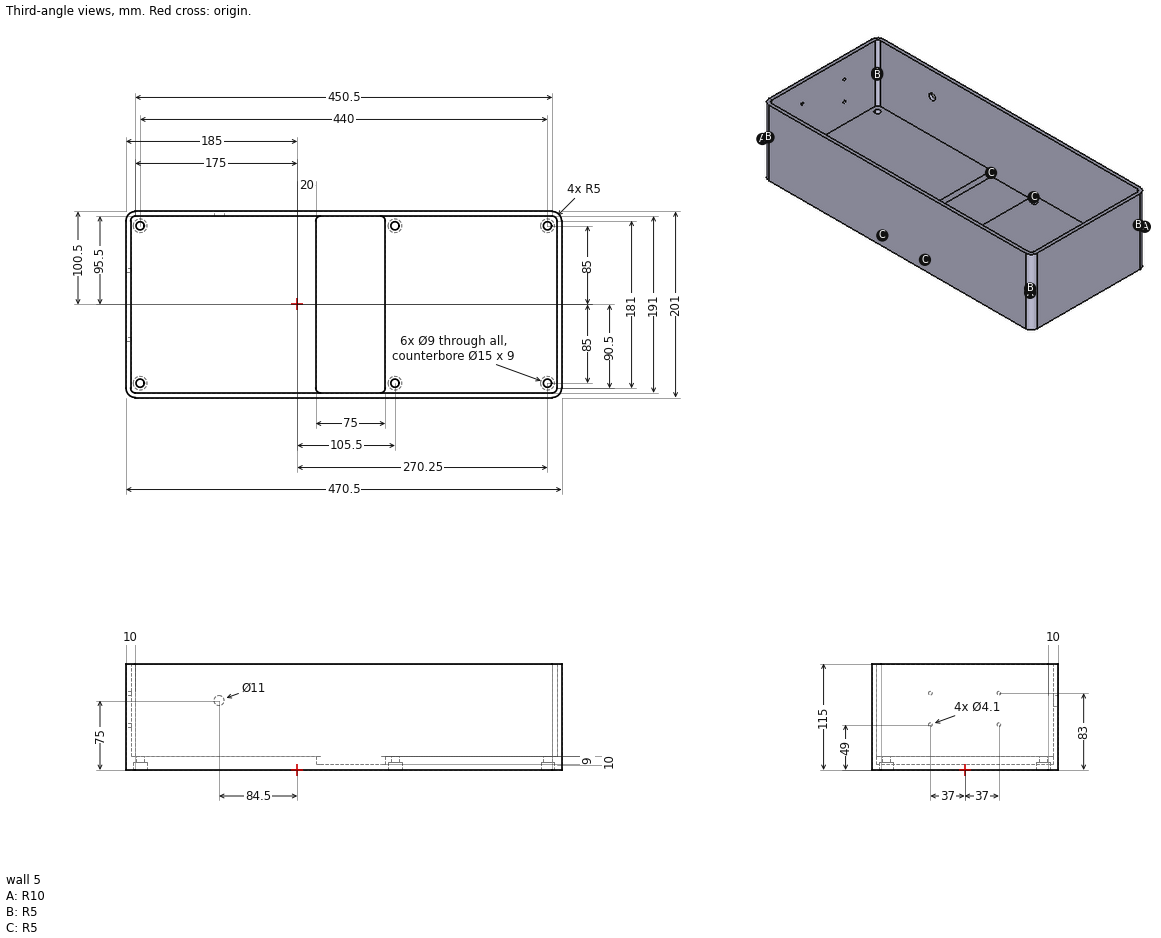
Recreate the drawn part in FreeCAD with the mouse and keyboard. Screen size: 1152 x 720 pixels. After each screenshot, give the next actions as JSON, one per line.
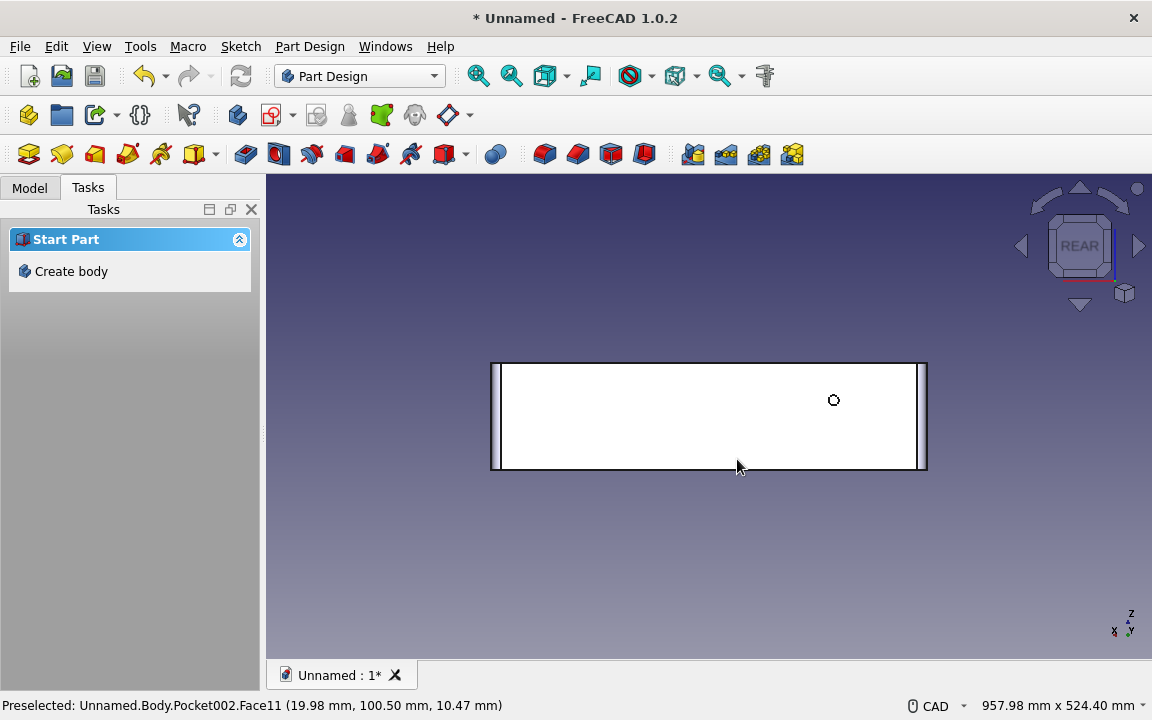
{"action": "key", "text": "6"}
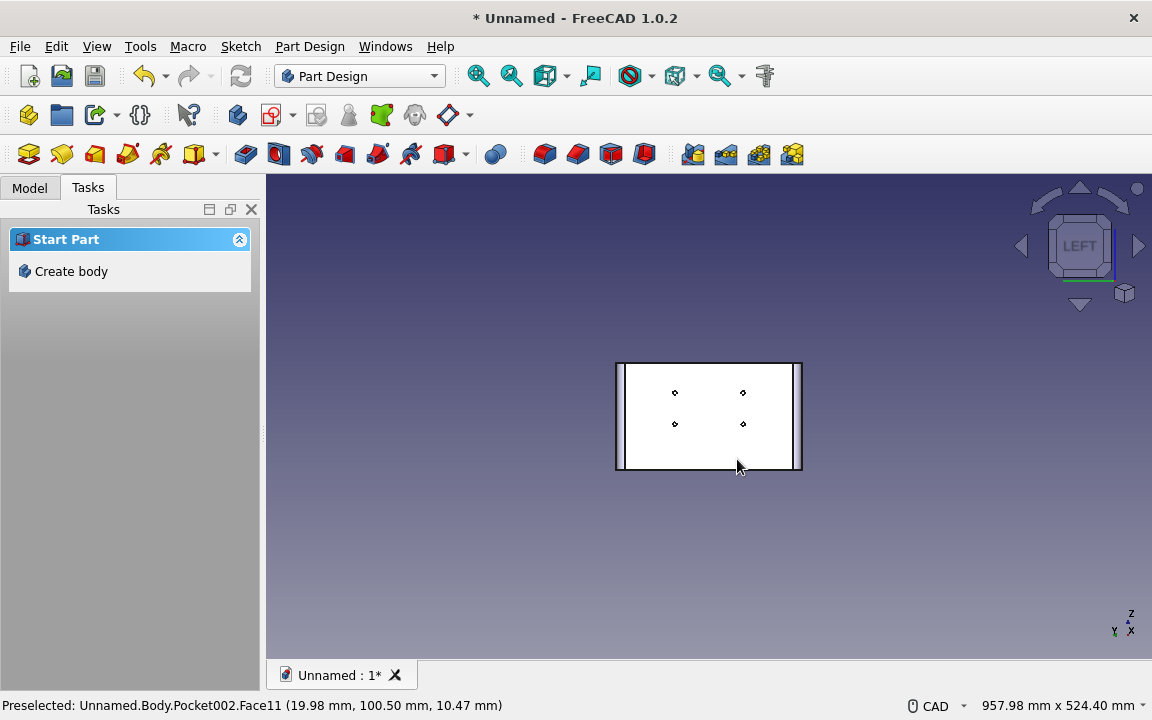
{"action": "key", "text": "v f"}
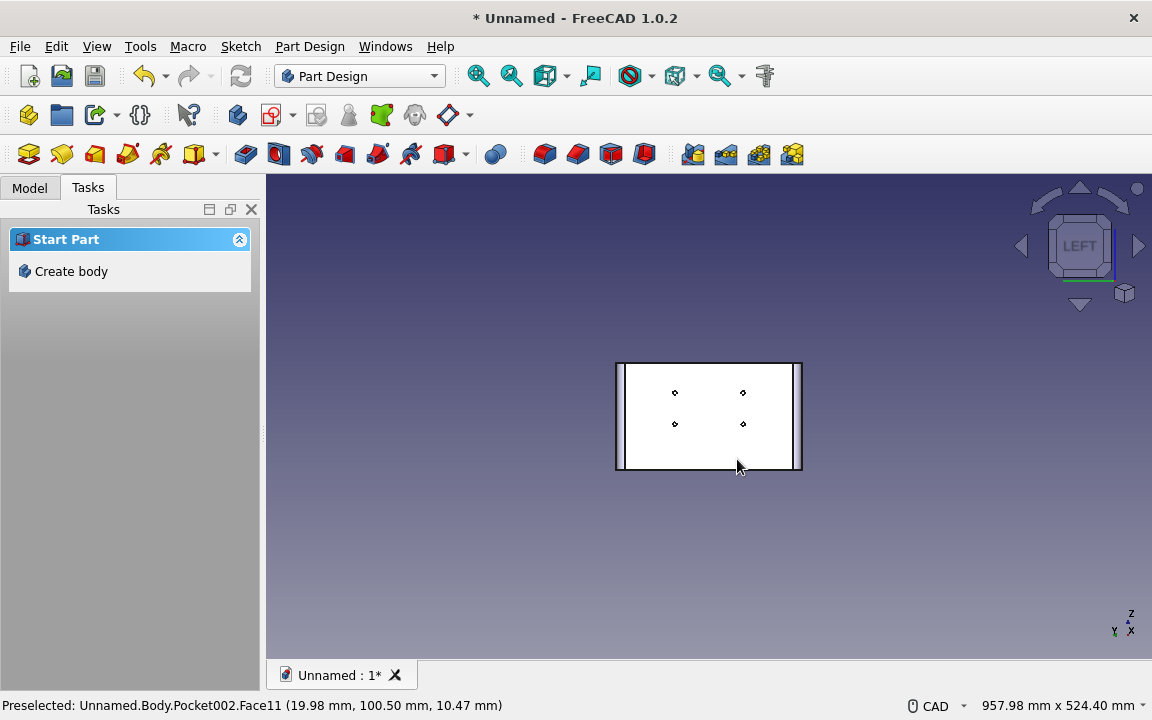
{"action": "scroll", "coordinate": [797, 459], "scroll_direction": "up", "scroll_amount": 8}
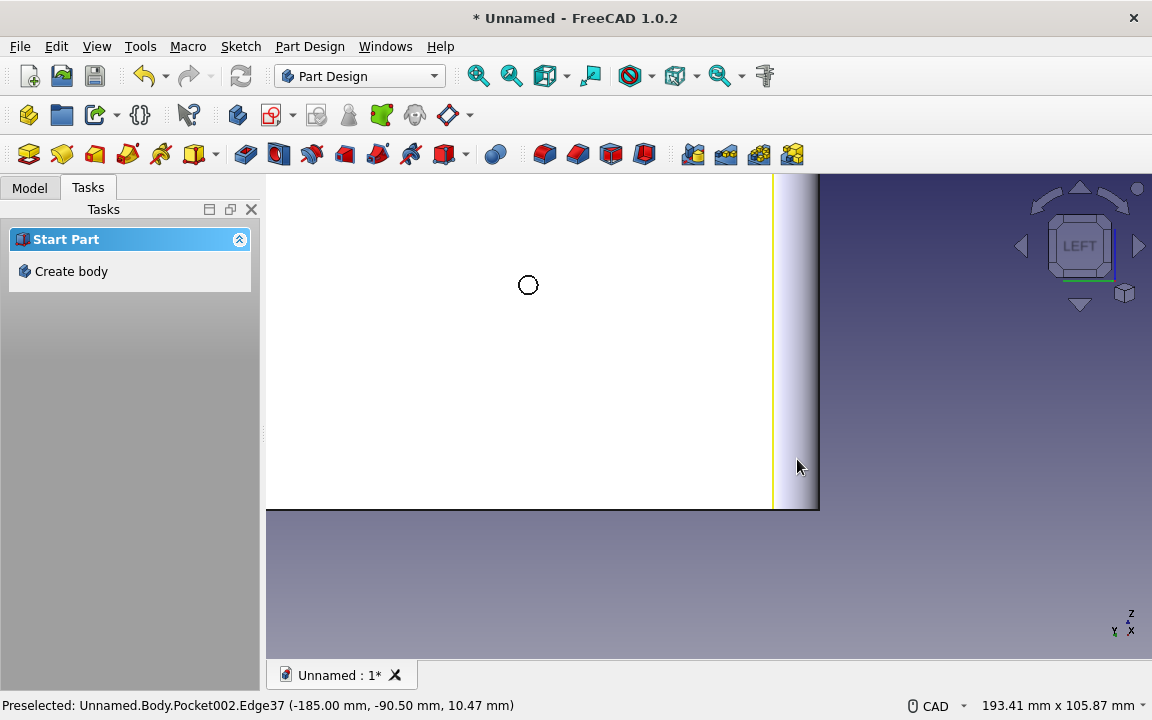
{"action": "key", "text": "v f"}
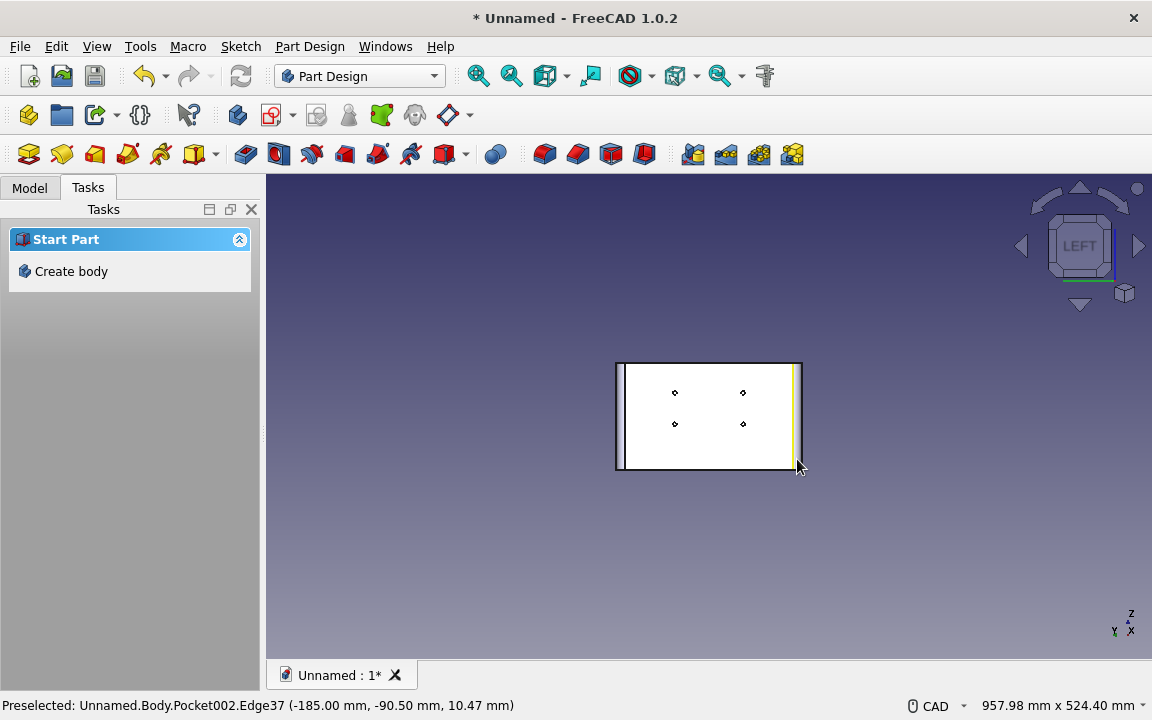
{"action": "key", "text": "v 3"}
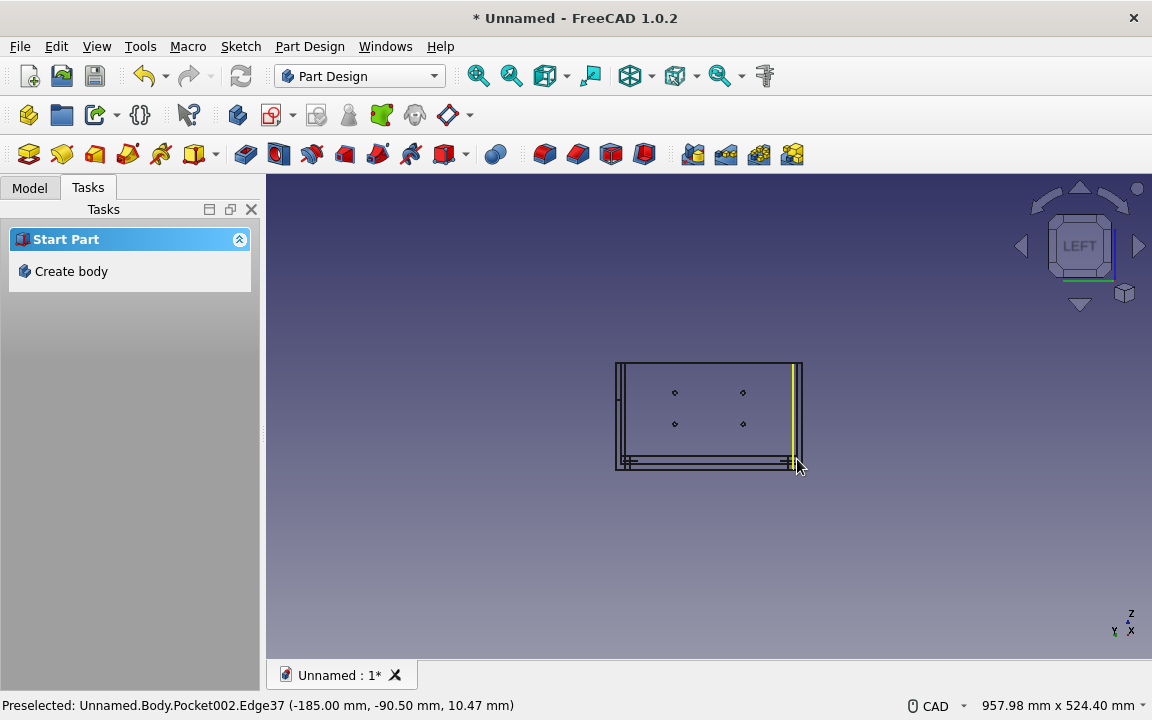
{"action": "key", "text": "0"}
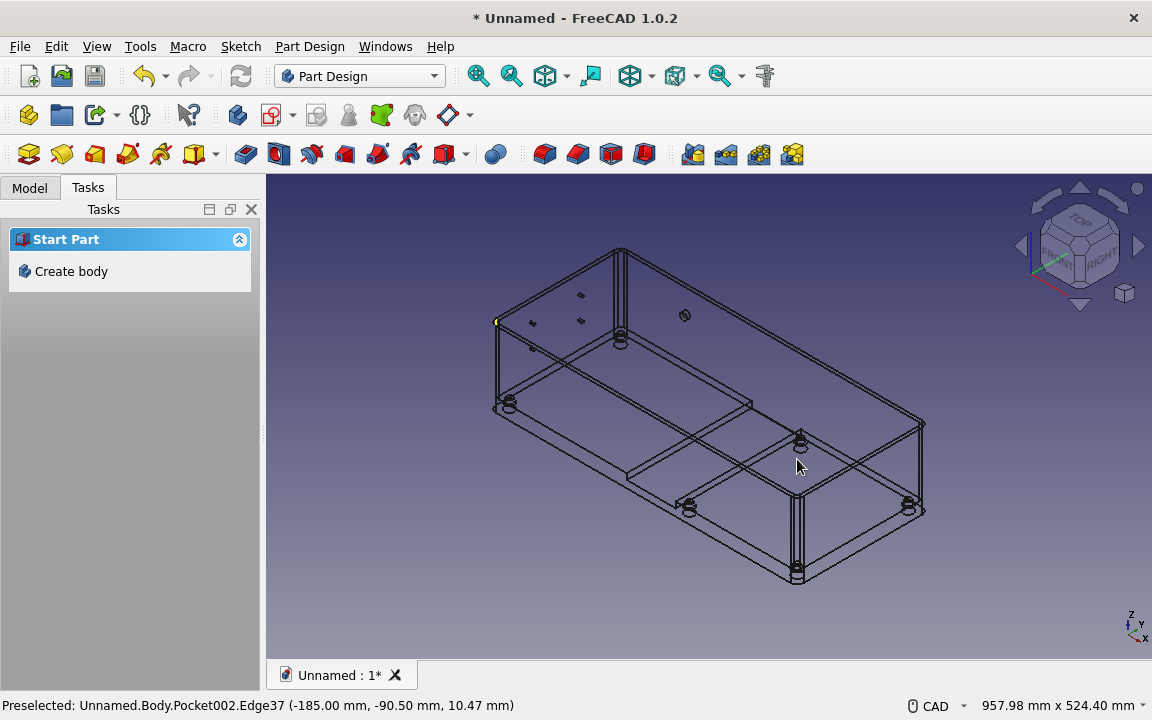
{"action": "scroll", "coordinate": [627, 476], "scroll_direction": "up", "scroll_amount": 8}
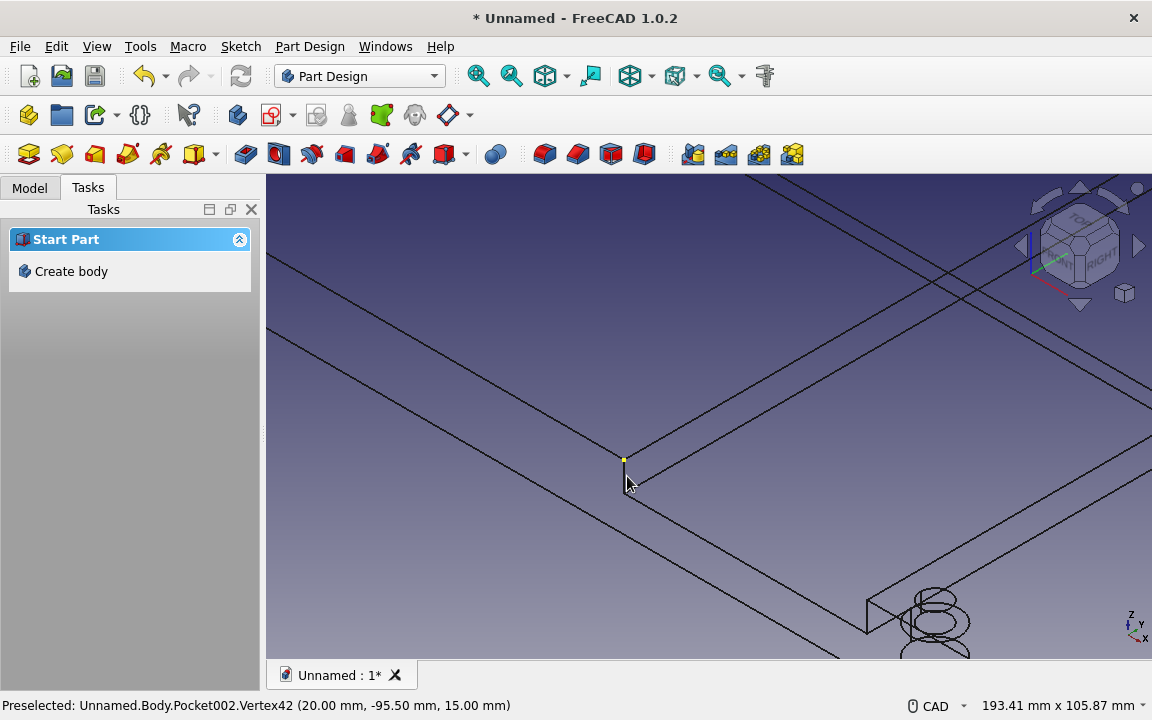
{"action": "left_click", "coordinate": [624, 476]}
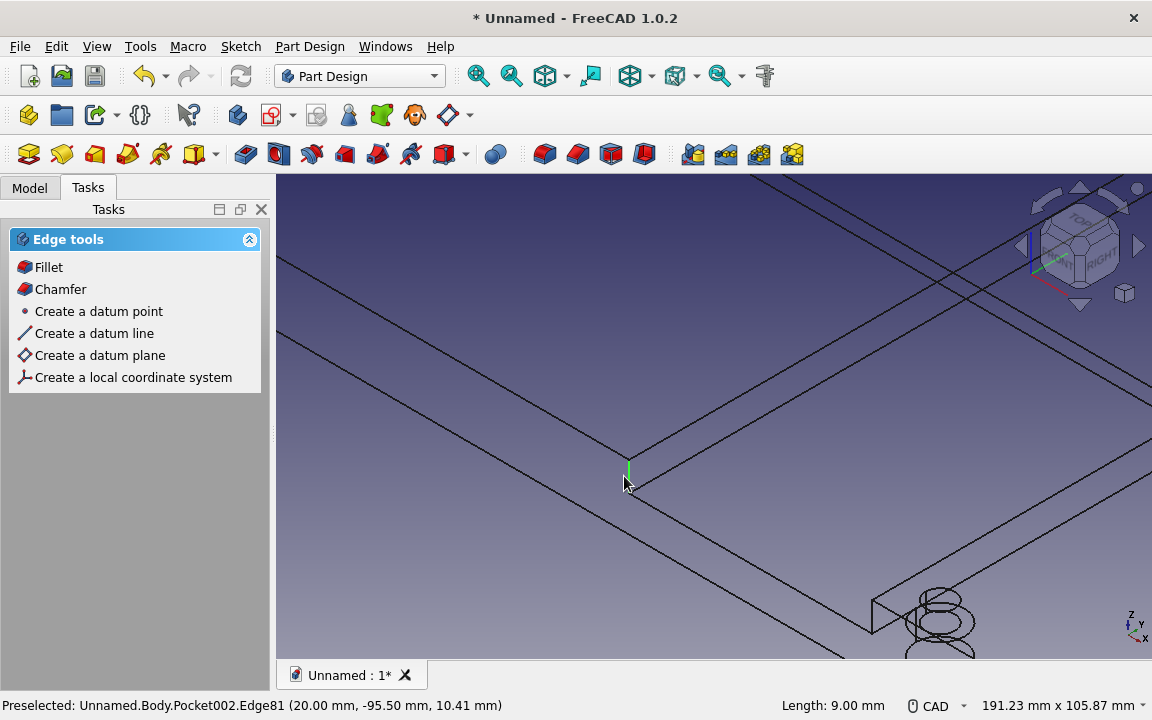
{"action": "left_click", "coordinate": [872, 616], "text": "ctrl"}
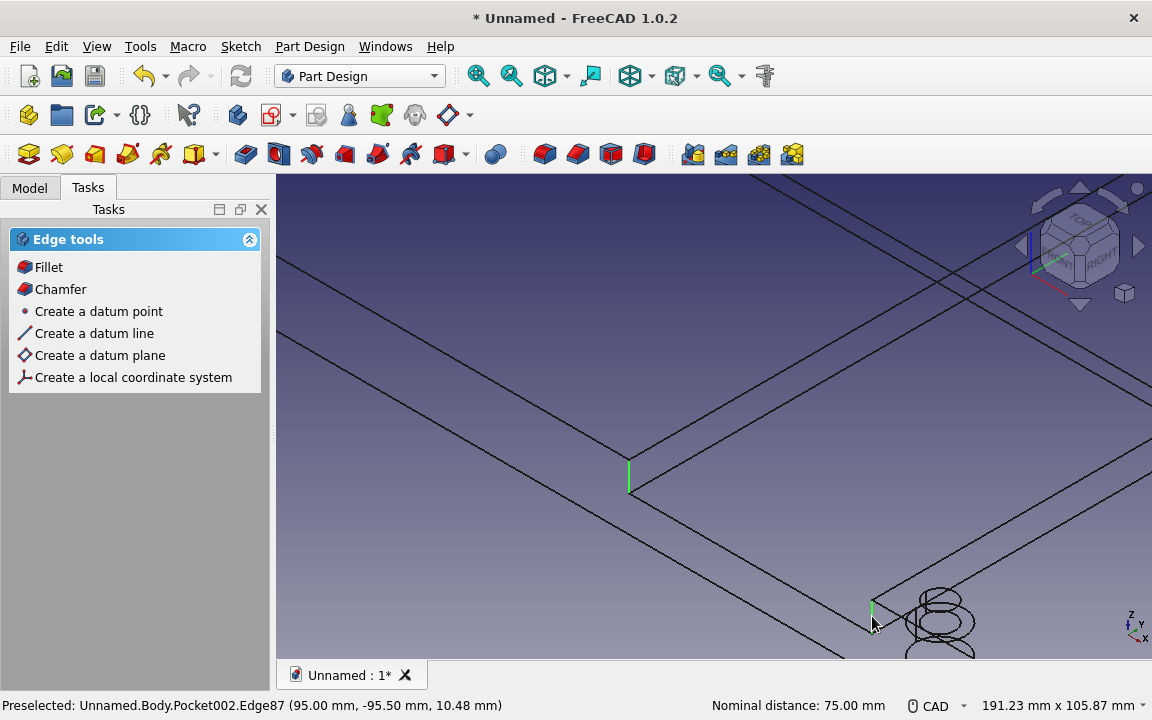
{"action": "key", "text": "v f"}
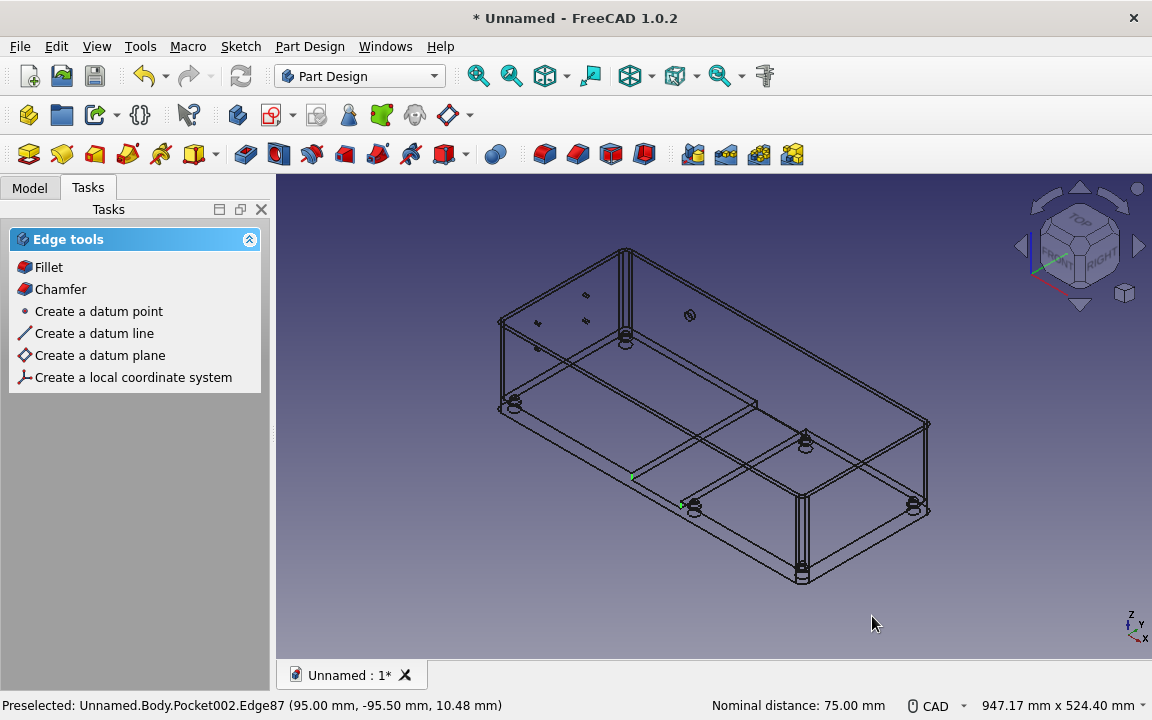
{"action": "key", "text": "2"}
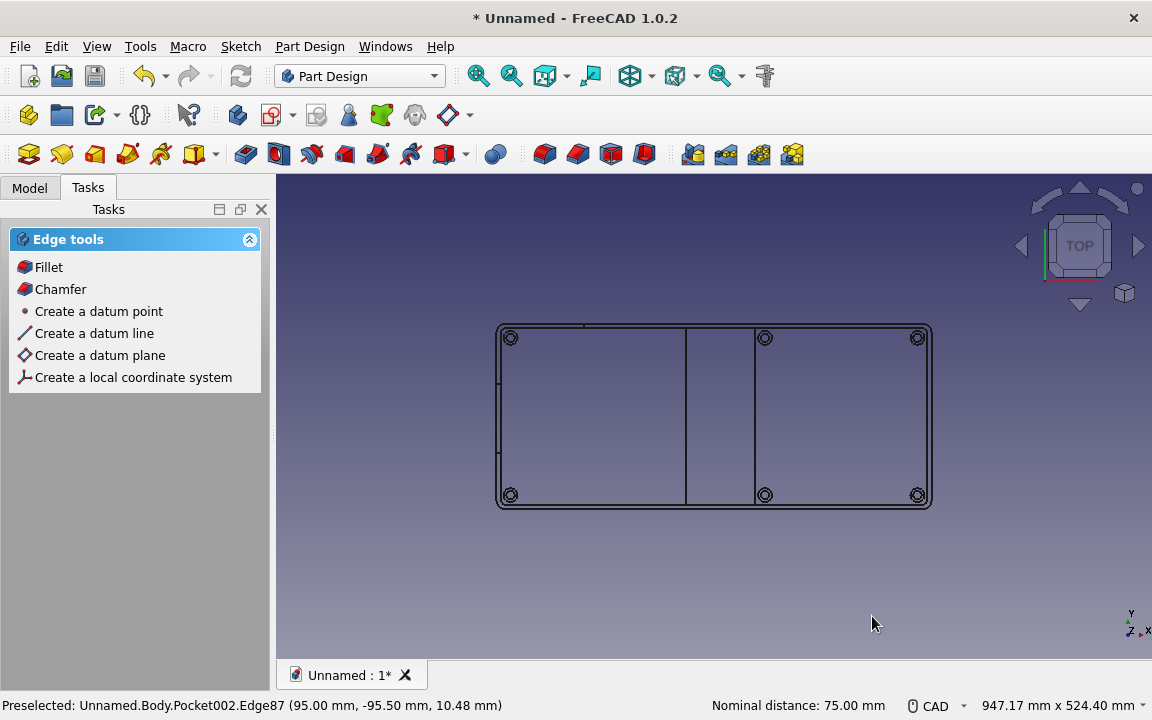
{"action": "scroll", "coordinate": [686, 327], "scroll_direction": "up", "scroll_amount": 8}